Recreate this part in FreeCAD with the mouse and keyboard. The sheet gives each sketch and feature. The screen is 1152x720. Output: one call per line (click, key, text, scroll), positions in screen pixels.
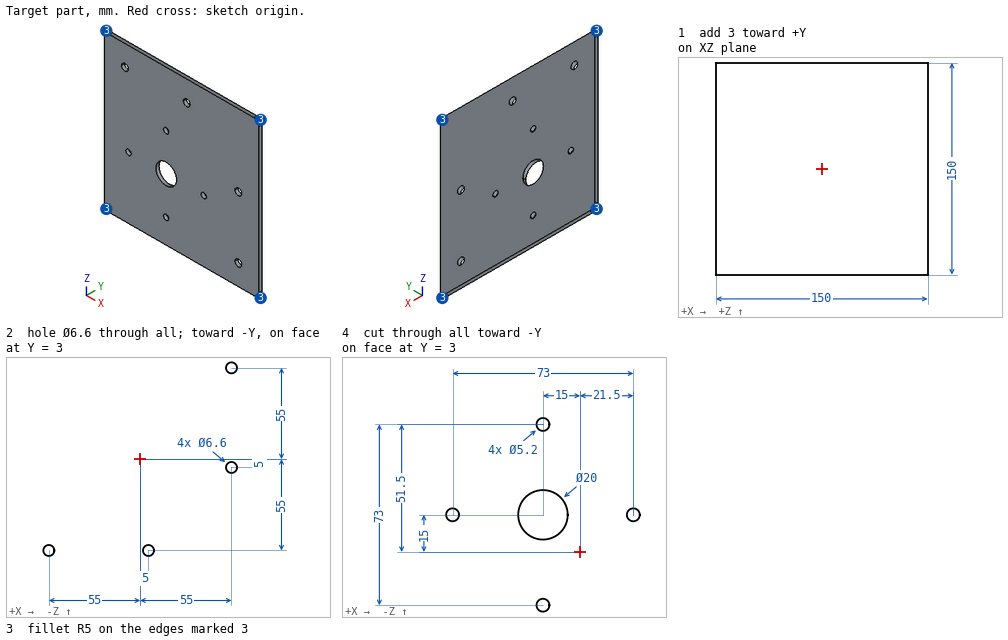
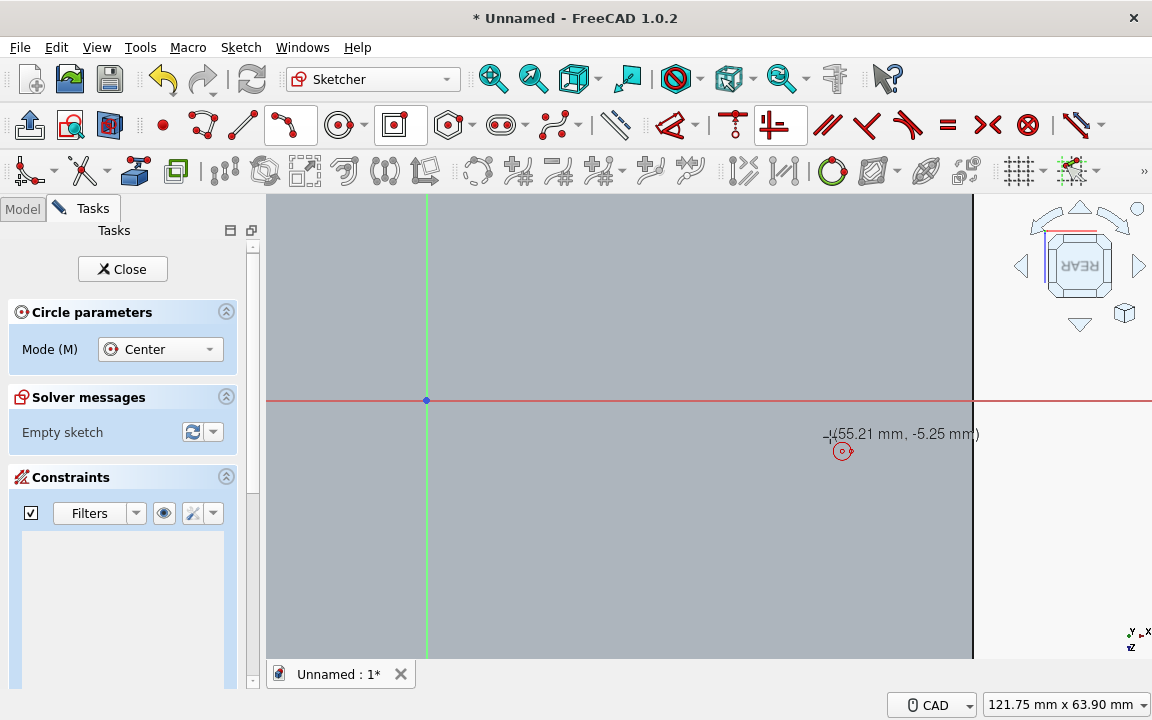
click(827, 437)
click(844, 420)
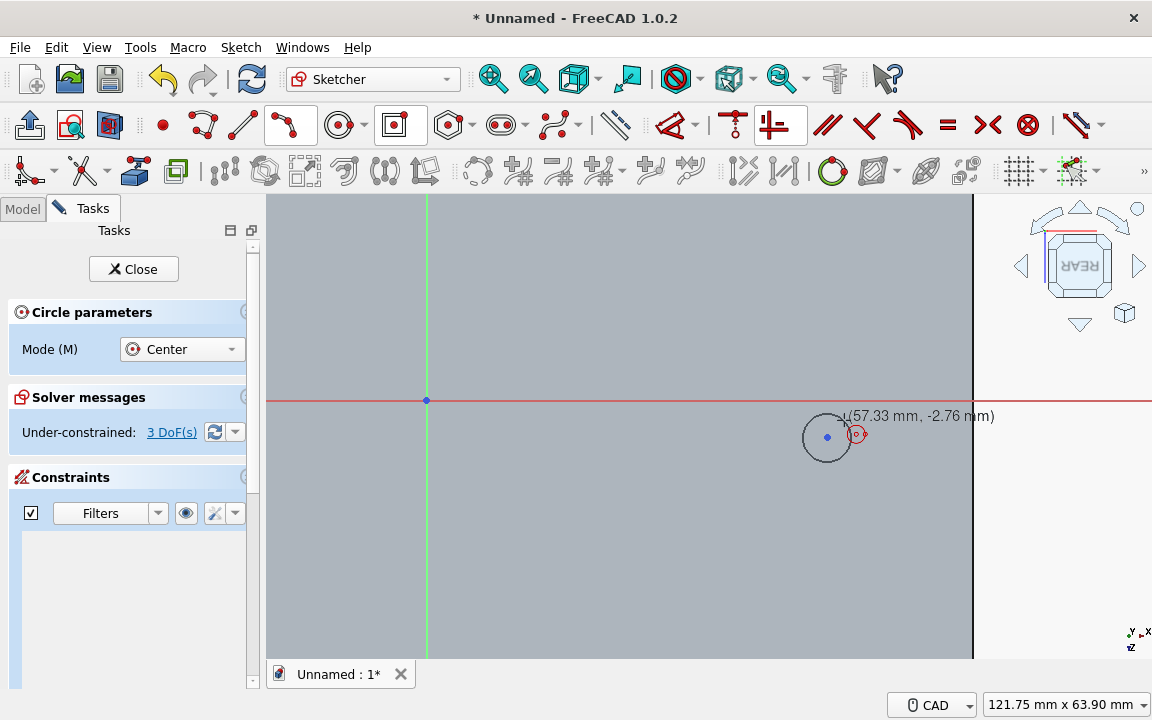
scroll(765, 441, down, 5)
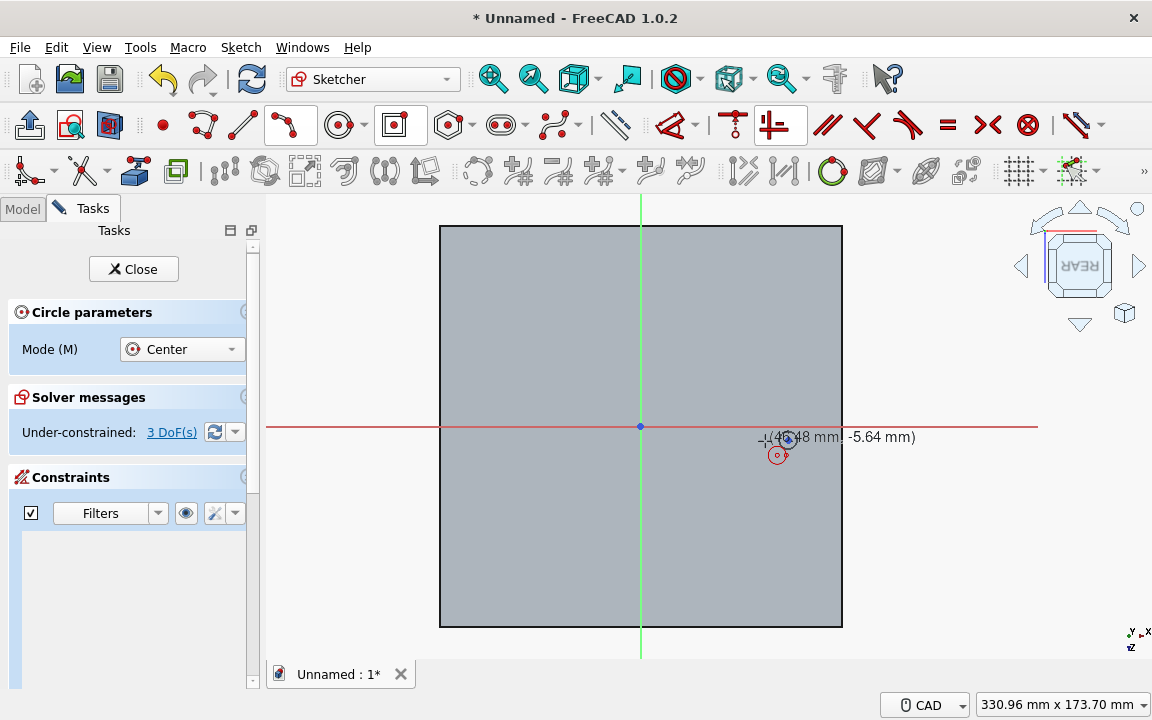
scroll(654, 574, up, 5)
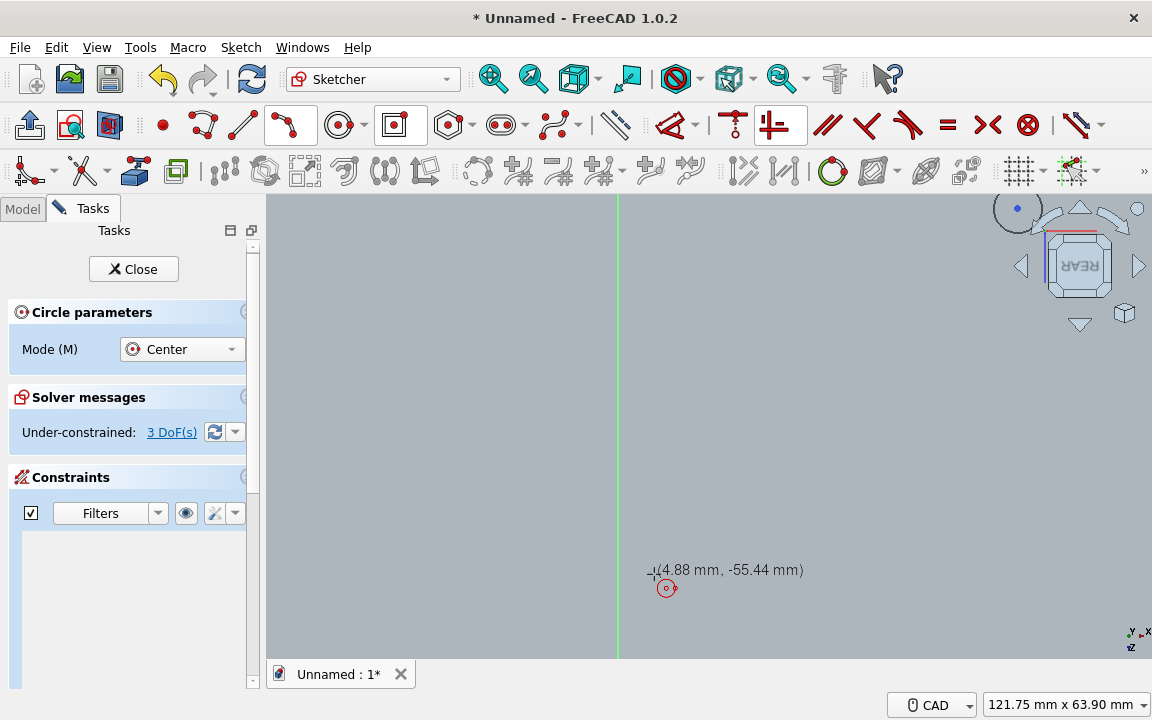
click(654, 572)
click(671, 555)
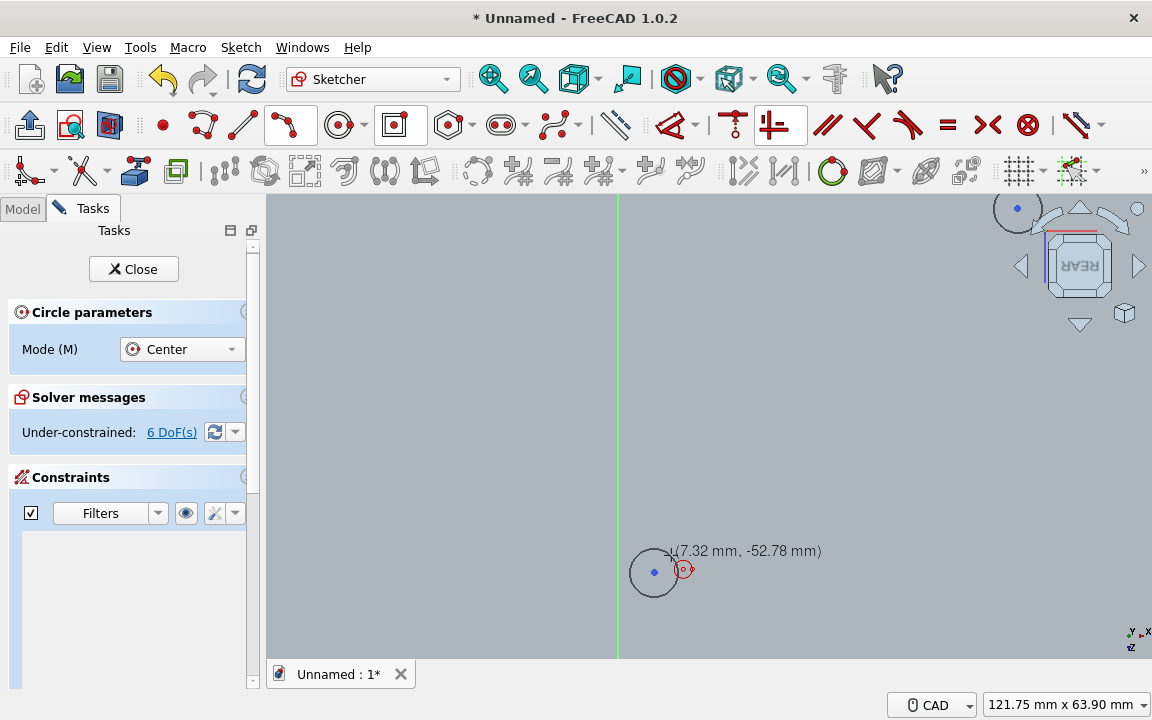
scroll(654, 575, down, 5)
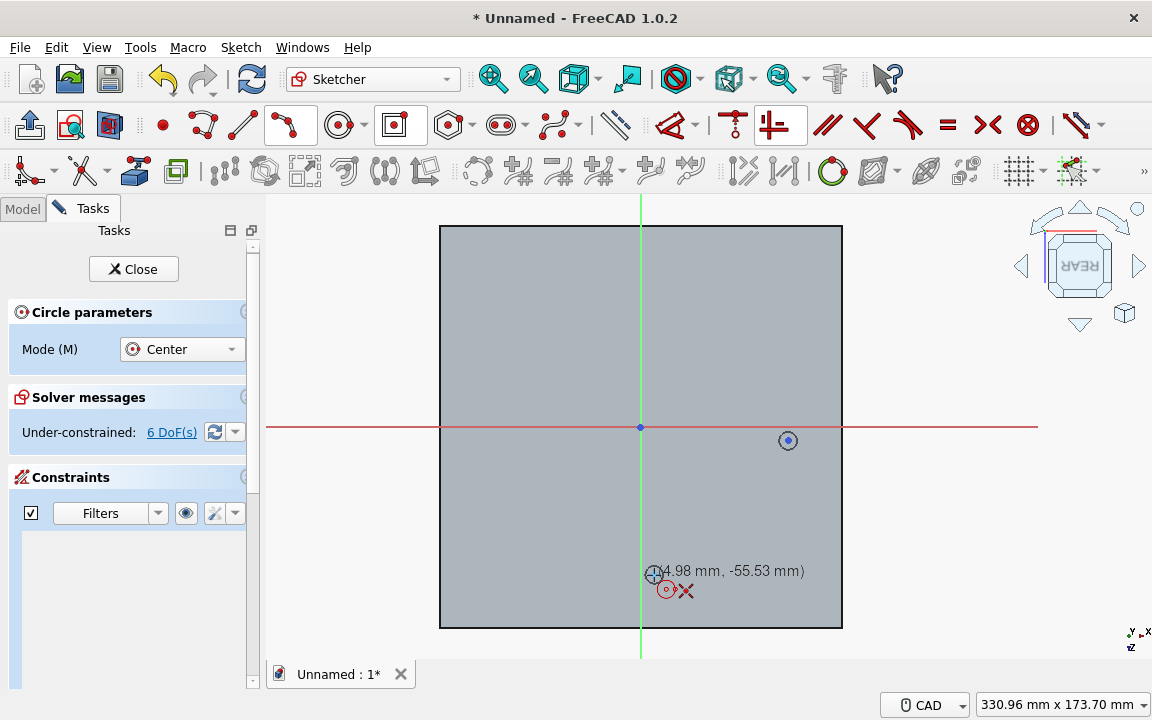
scroll(494, 574, up, 5)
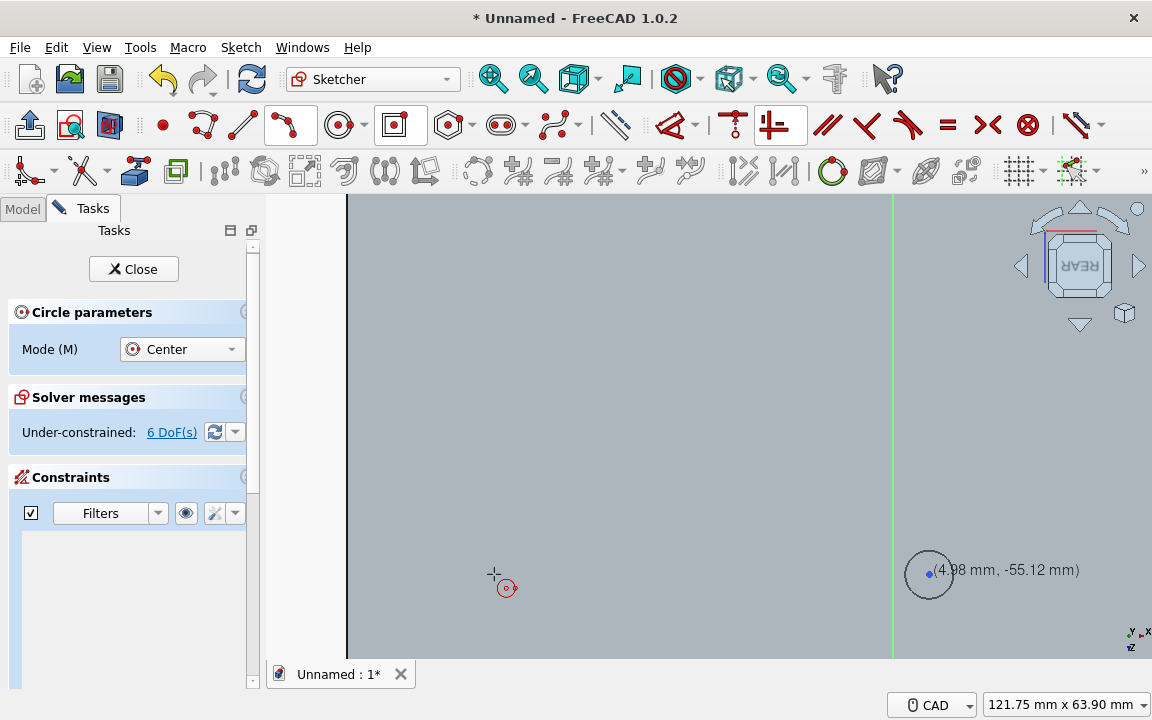
click(493, 574)
click(510, 557)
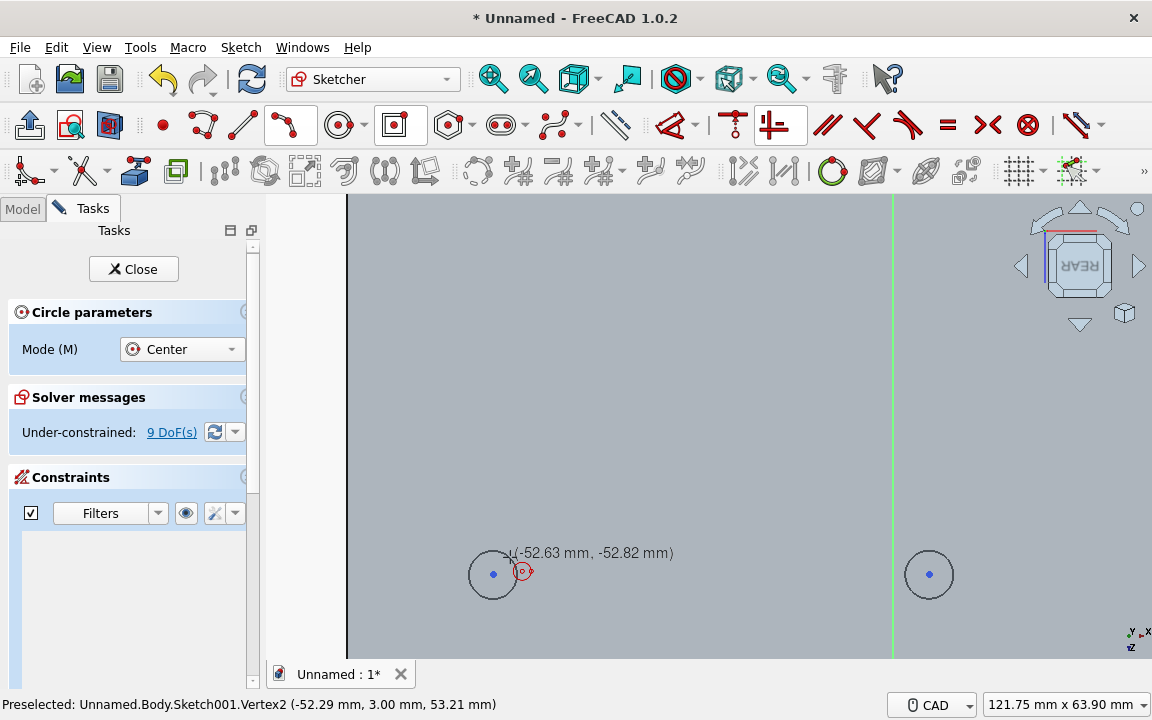
scroll(494, 574, down, 5)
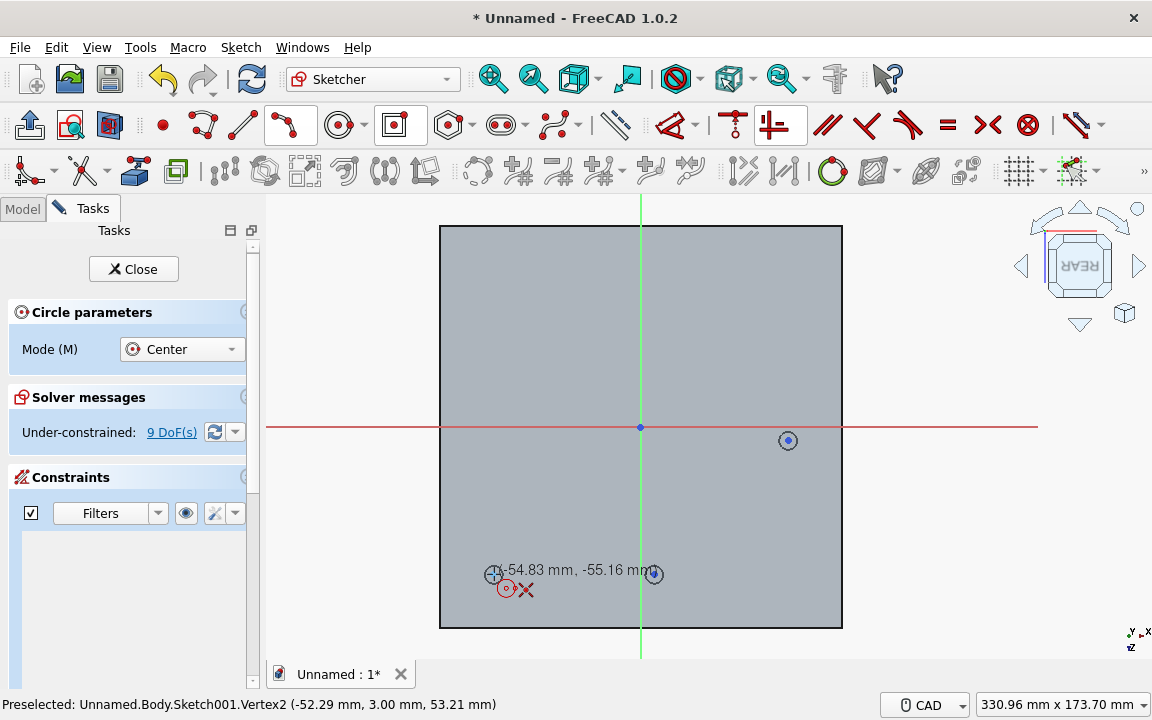
scroll(788, 280, up, 5)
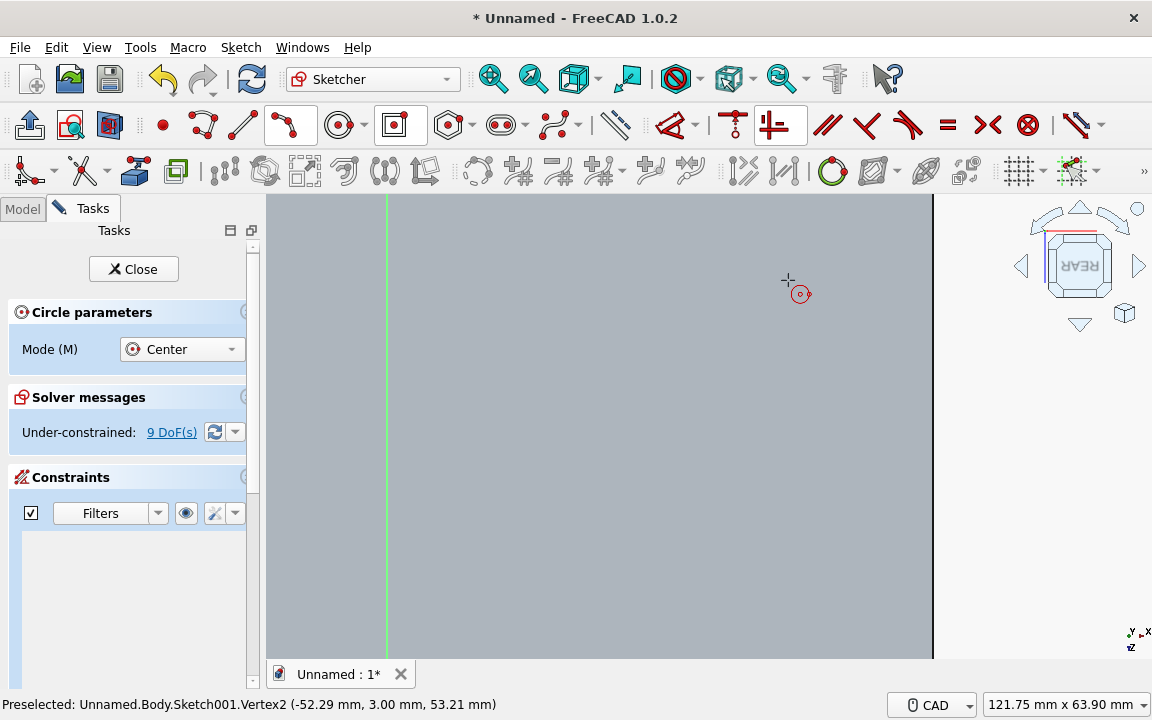
click(787, 280)
click(804, 263)
key(Escape)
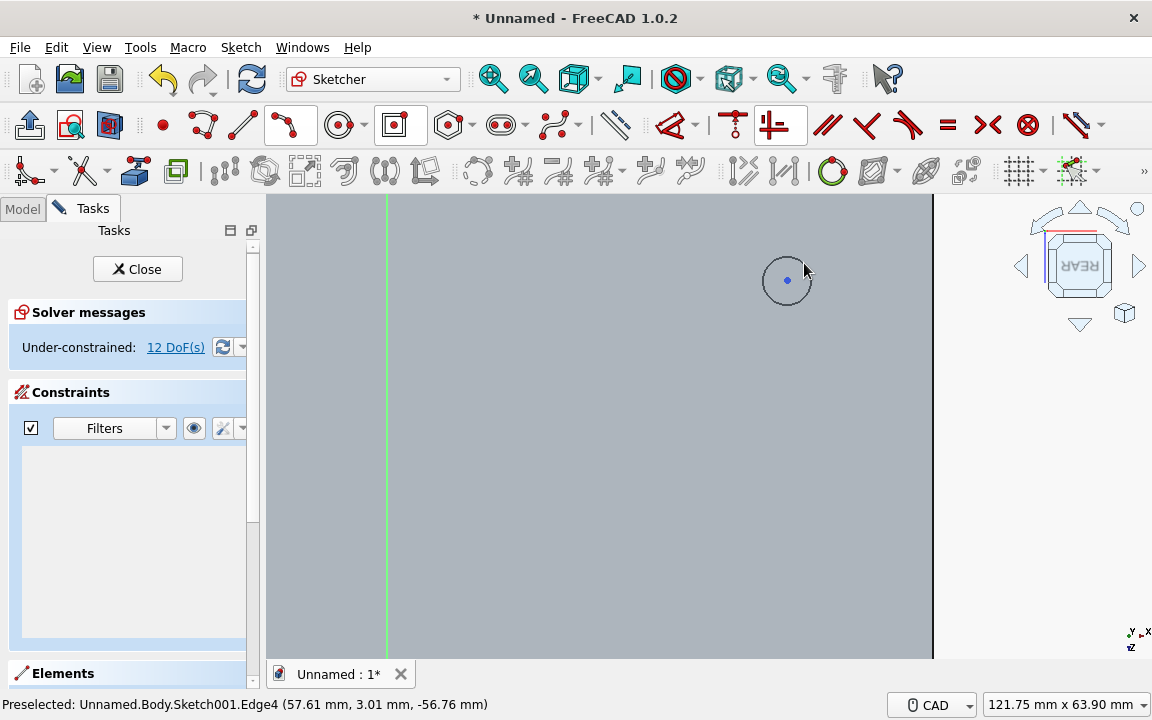
scroll(788, 279, down, 5)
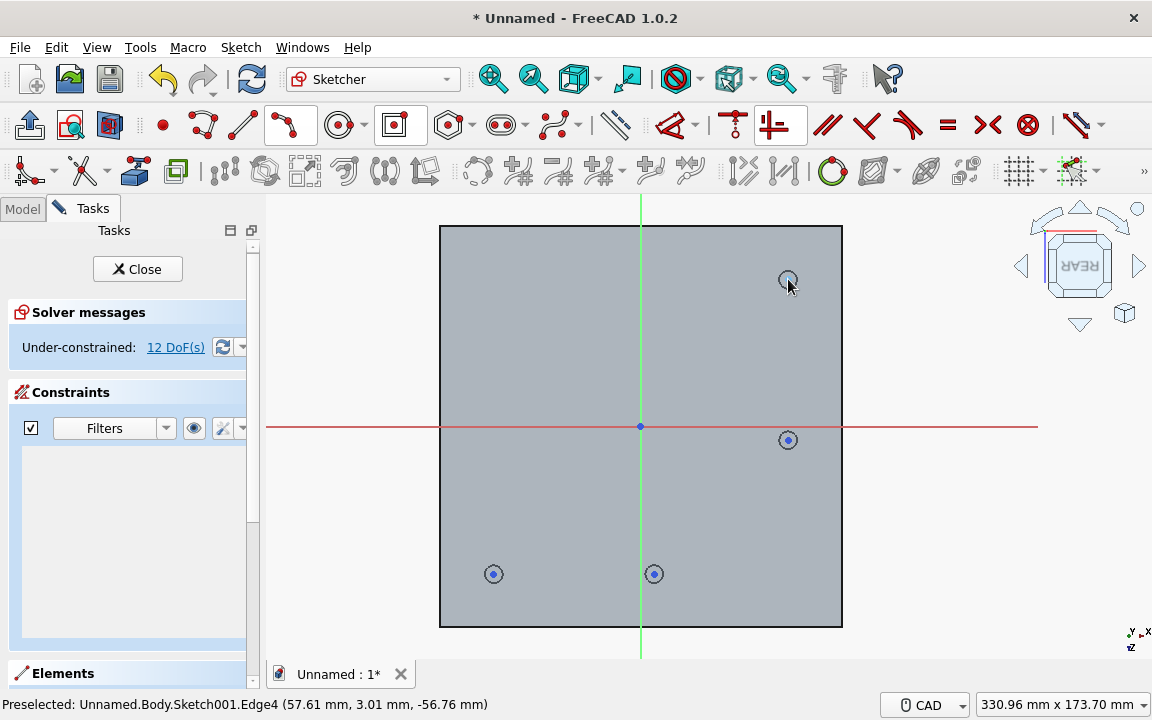
scroll(794, 434, up, 4)